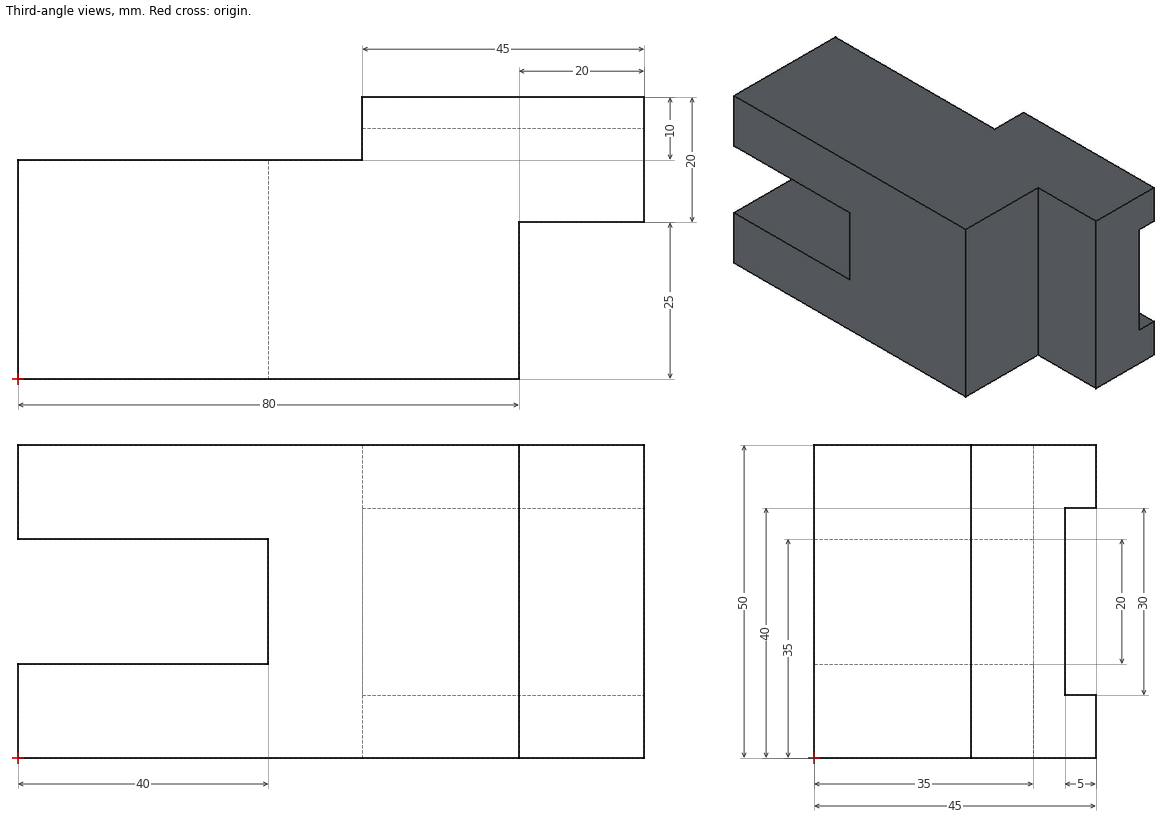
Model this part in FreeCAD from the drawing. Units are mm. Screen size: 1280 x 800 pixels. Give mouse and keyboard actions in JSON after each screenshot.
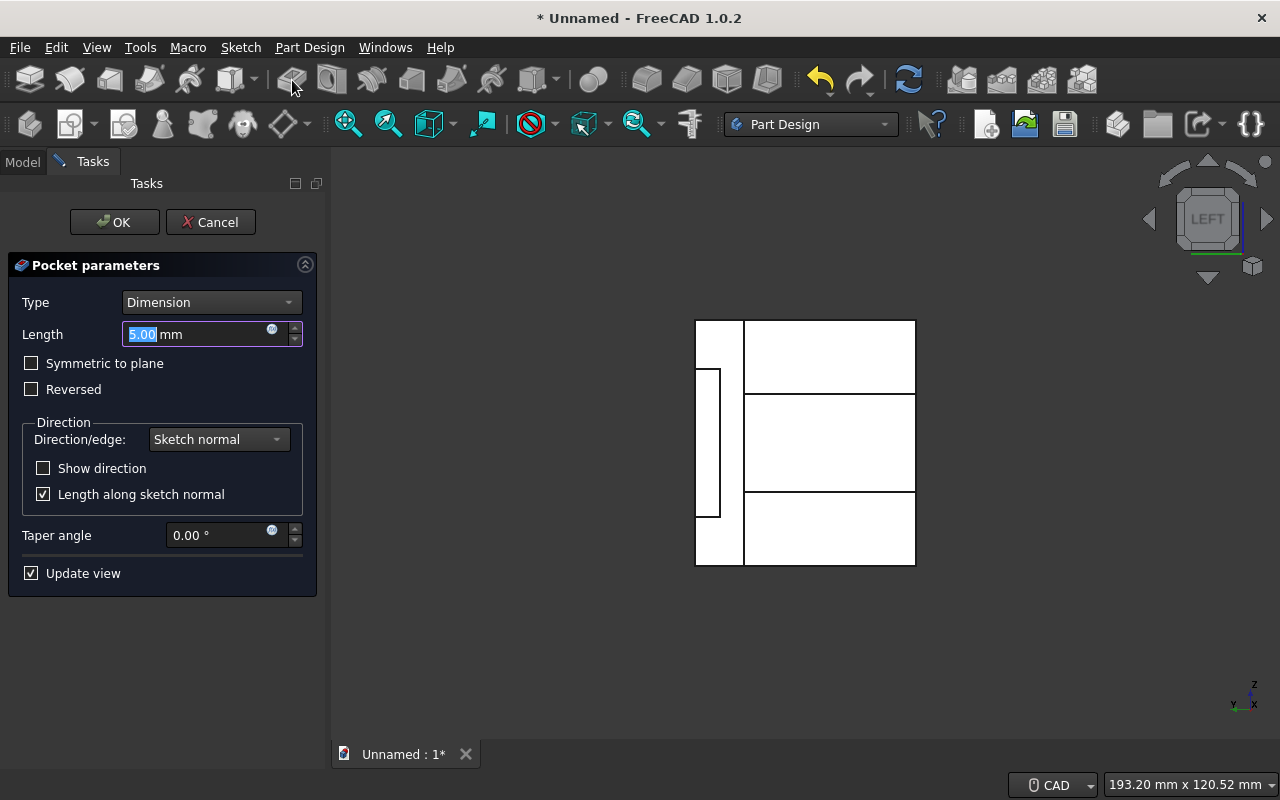
{"action": "left_click", "coordinate": [212, 302]}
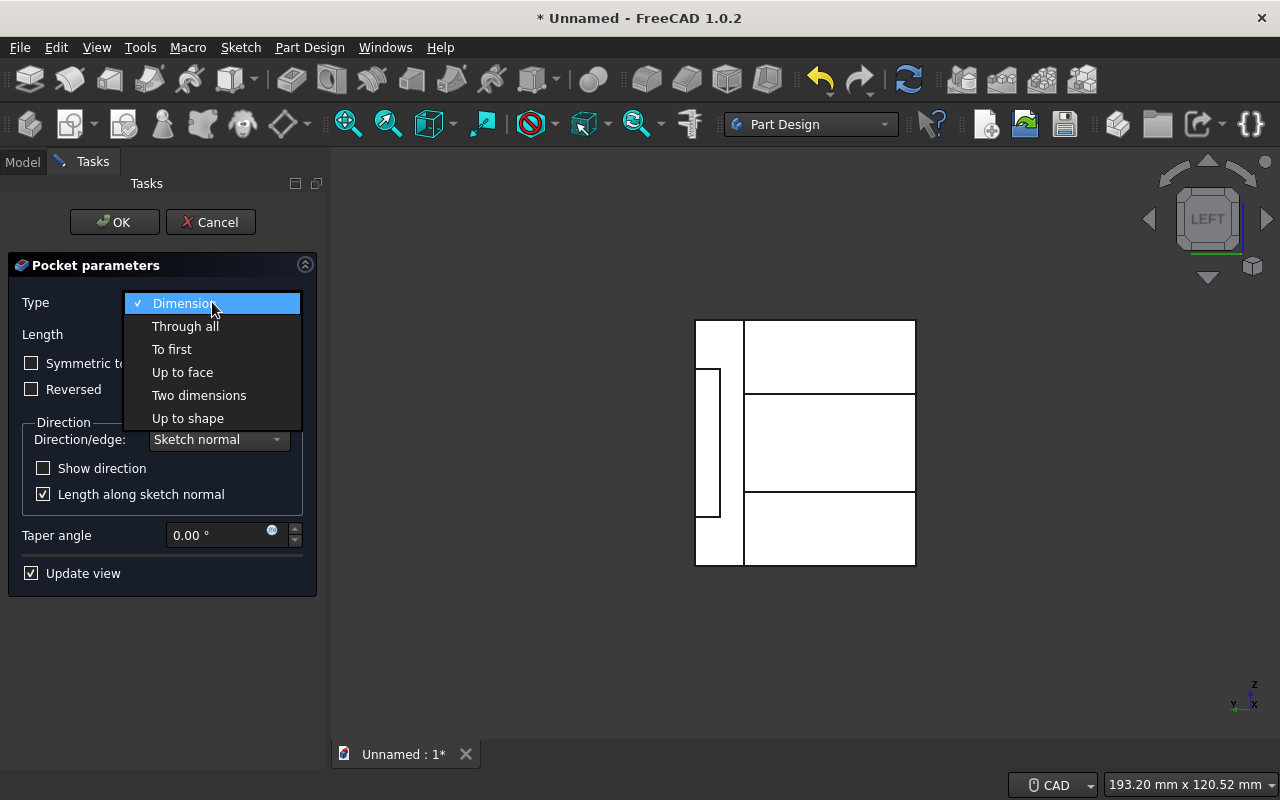
{"action": "left_click", "coordinate": [212, 326]}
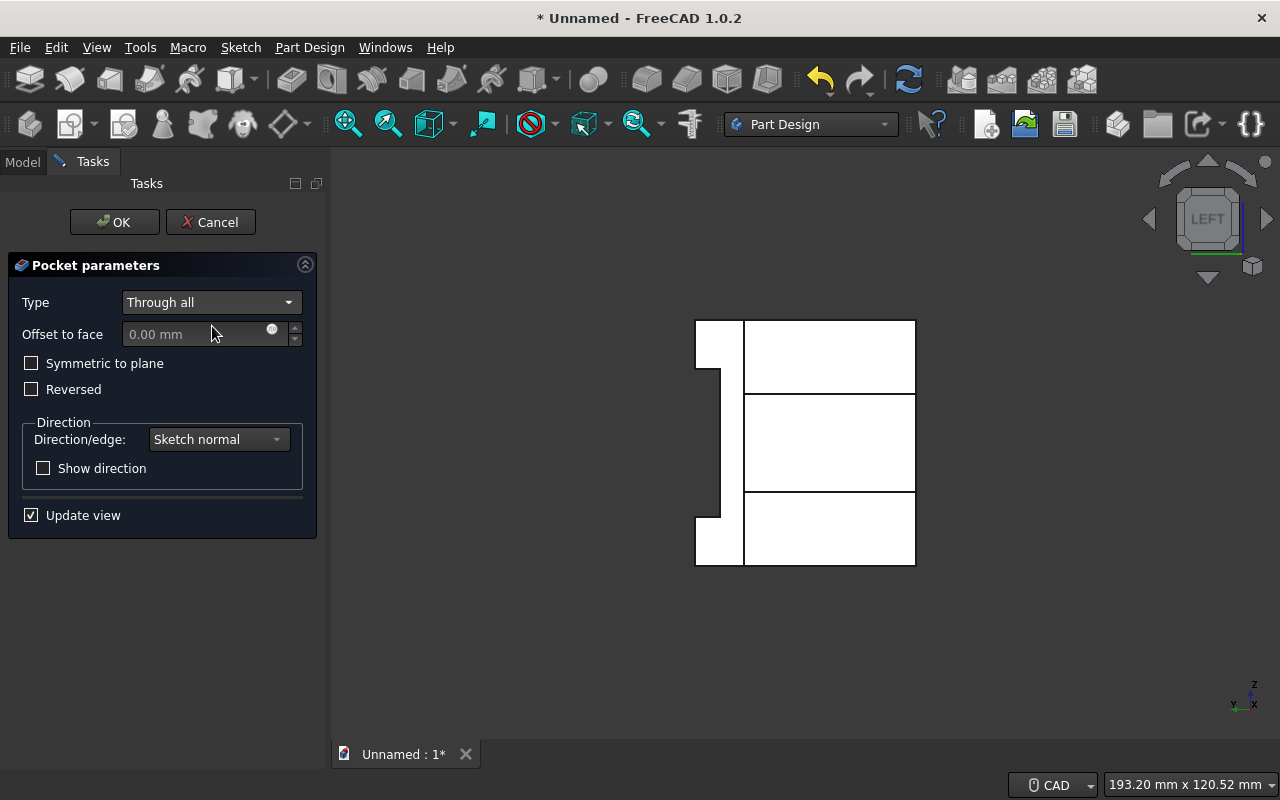
{"action": "left_click", "coordinate": [115, 222]}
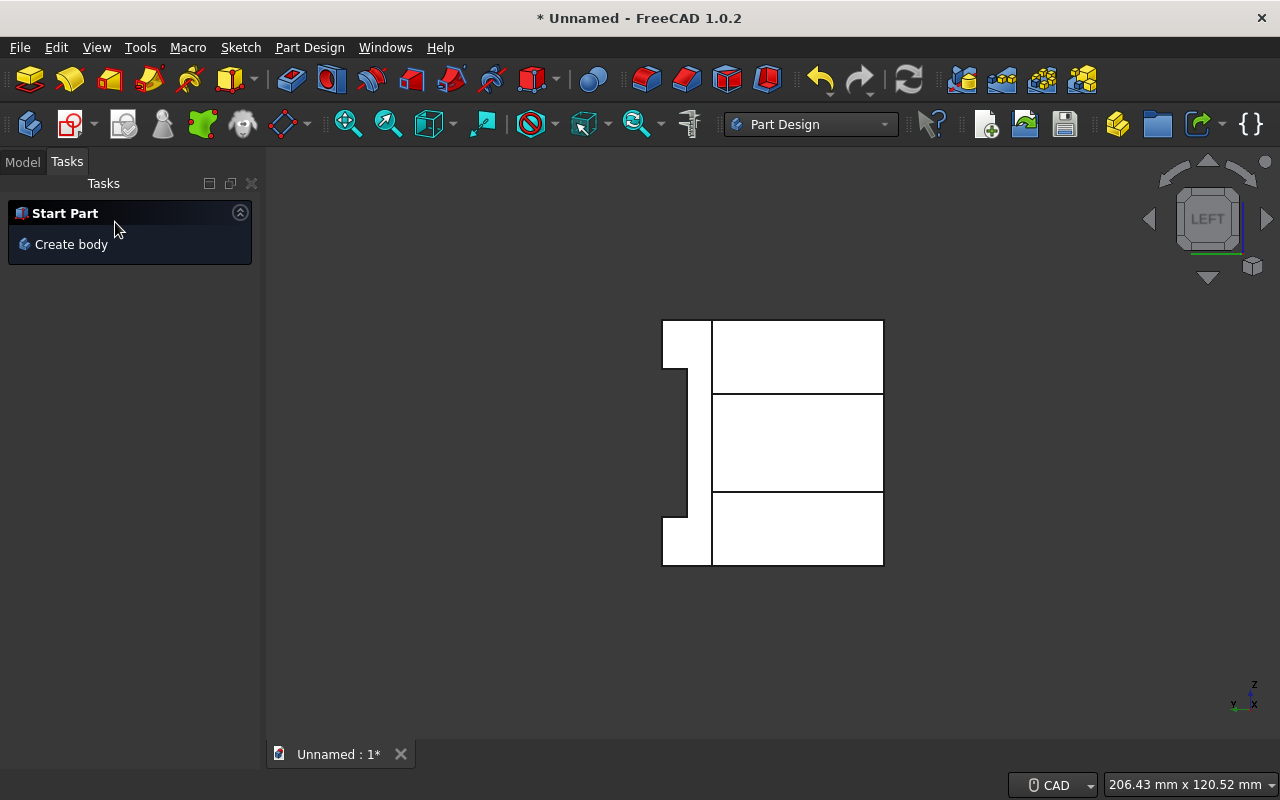
{"action": "key", "text": "0"}